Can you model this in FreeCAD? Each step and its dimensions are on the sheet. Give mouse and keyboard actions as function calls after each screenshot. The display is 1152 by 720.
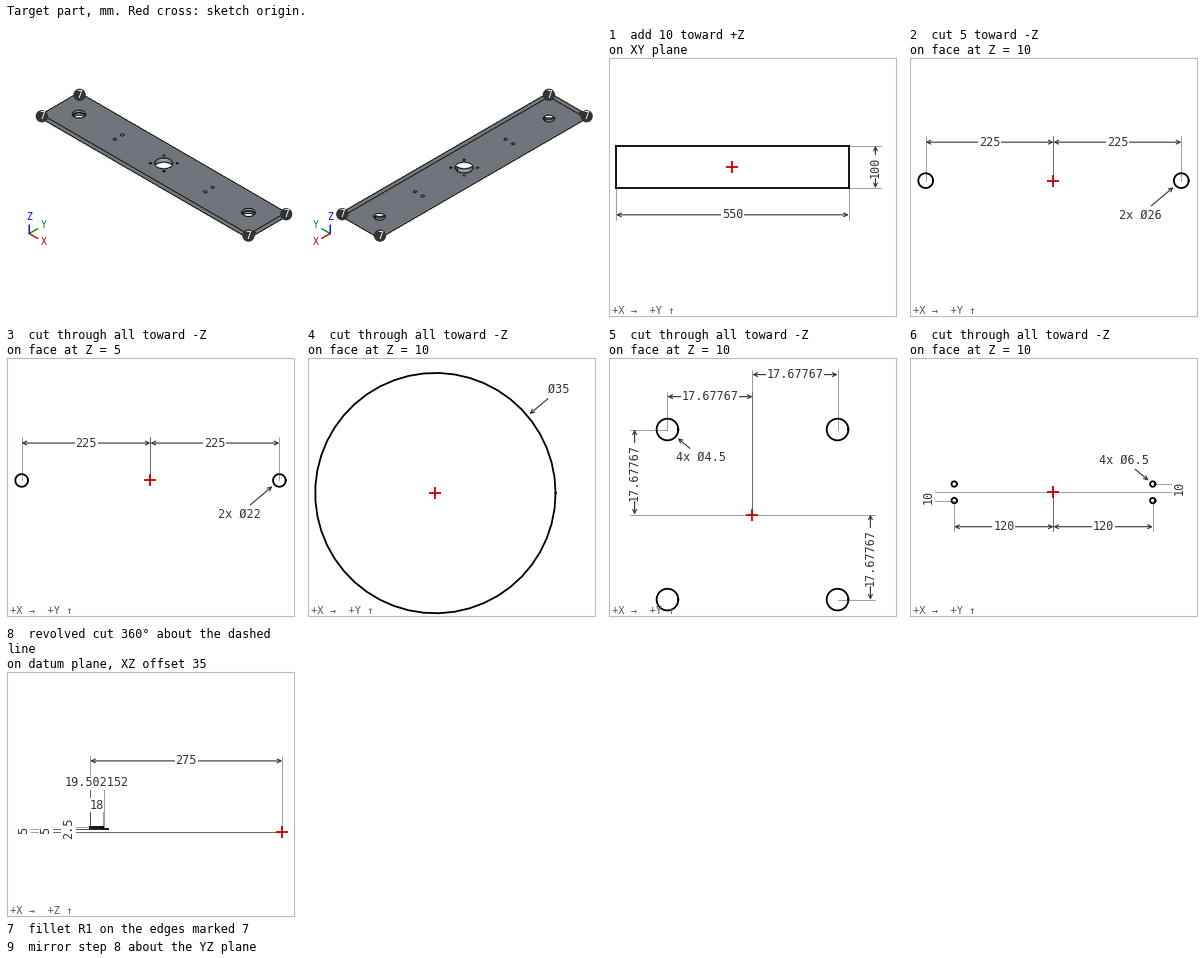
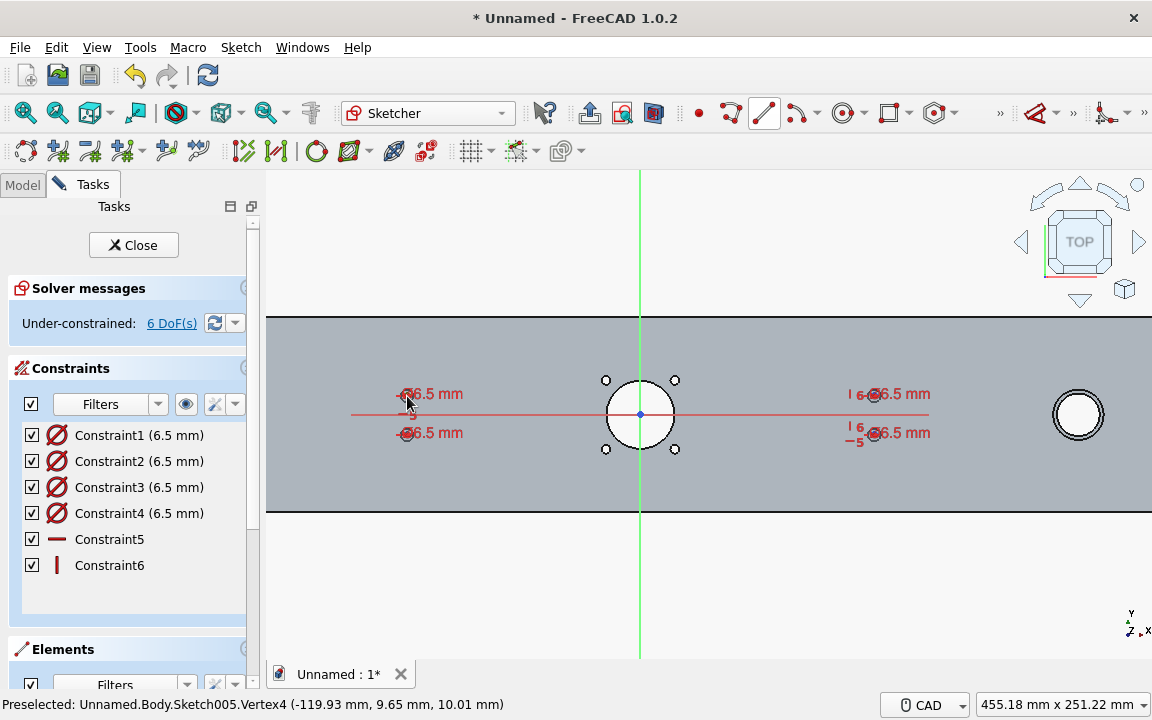
key(v)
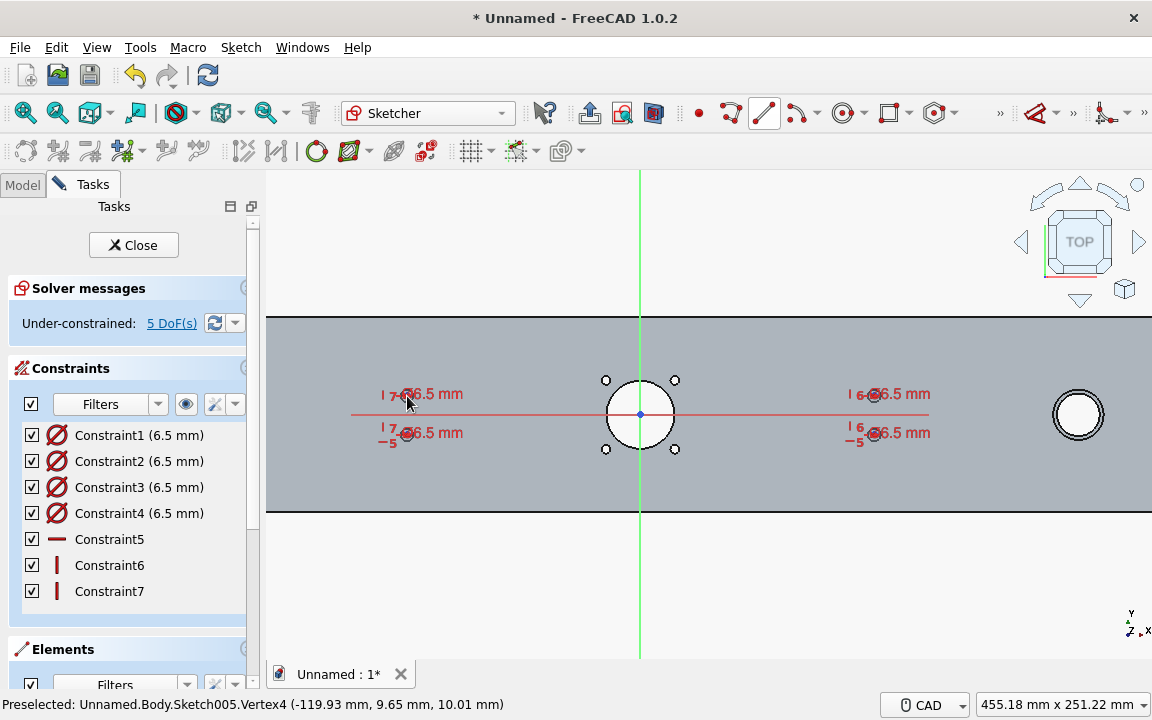
click(874, 396)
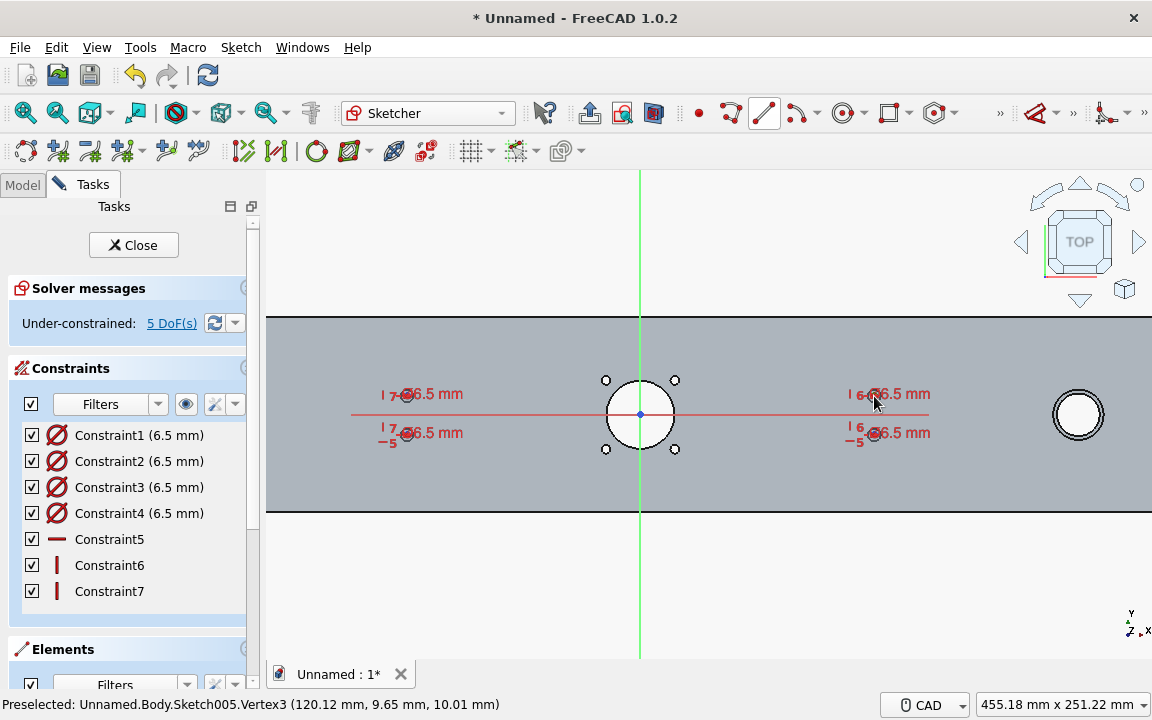
click(407, 396)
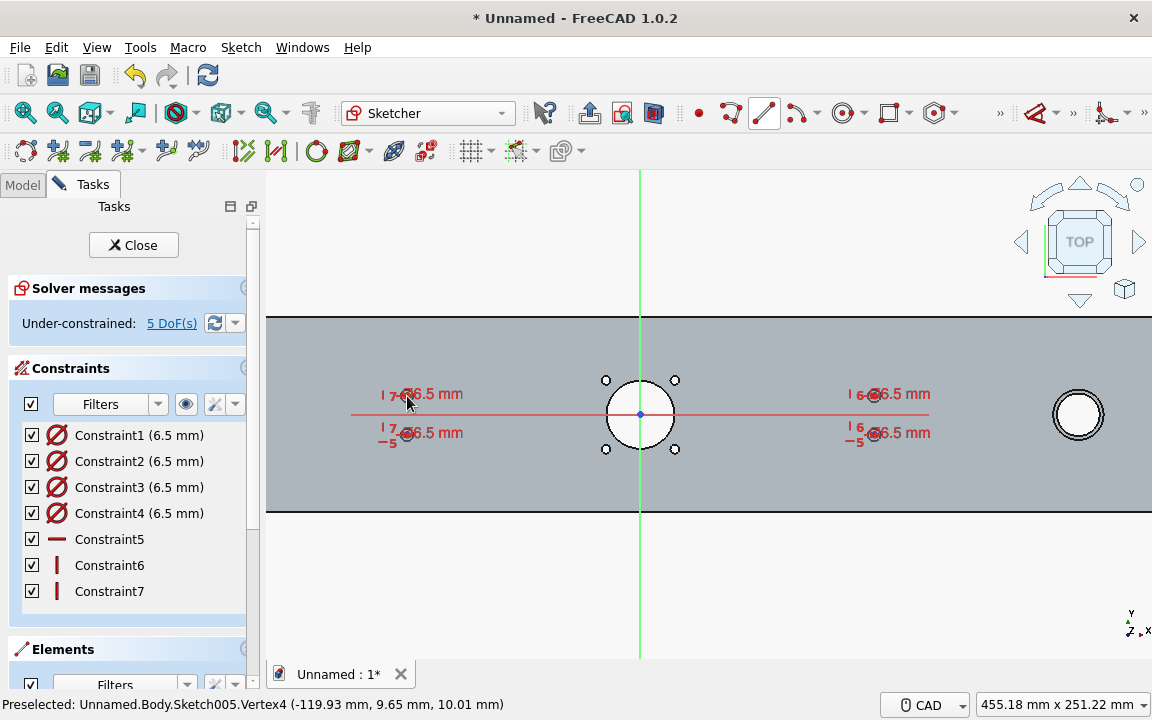
key(h)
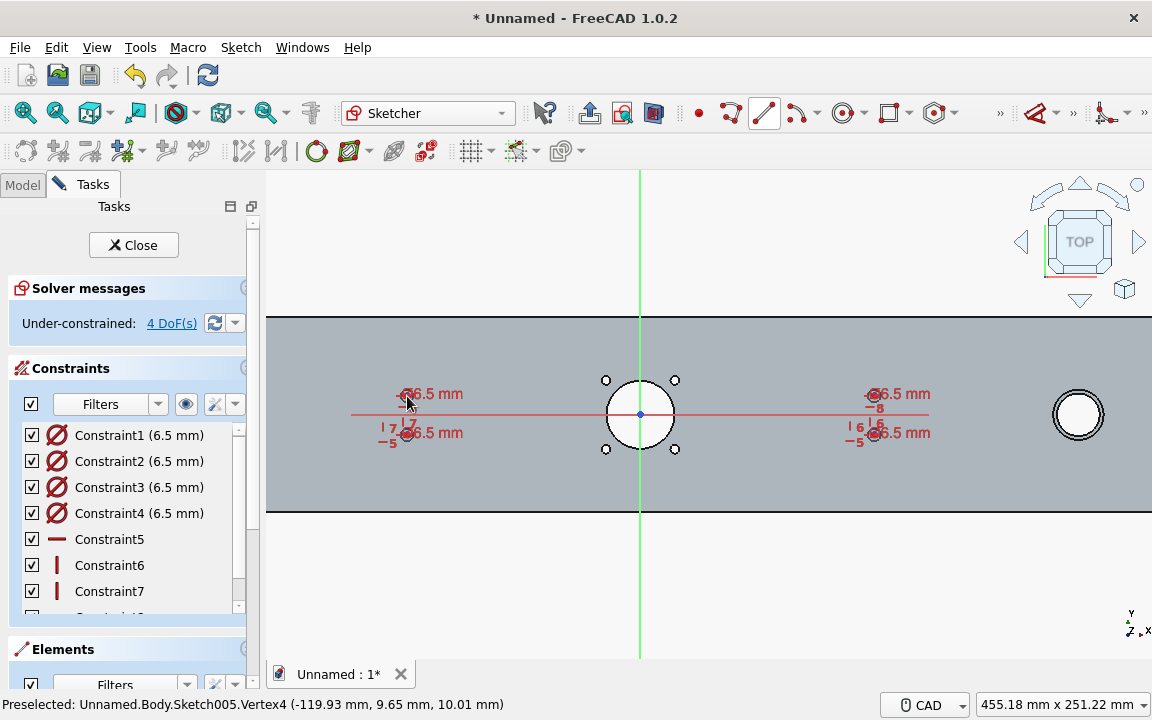
click(1036, 114)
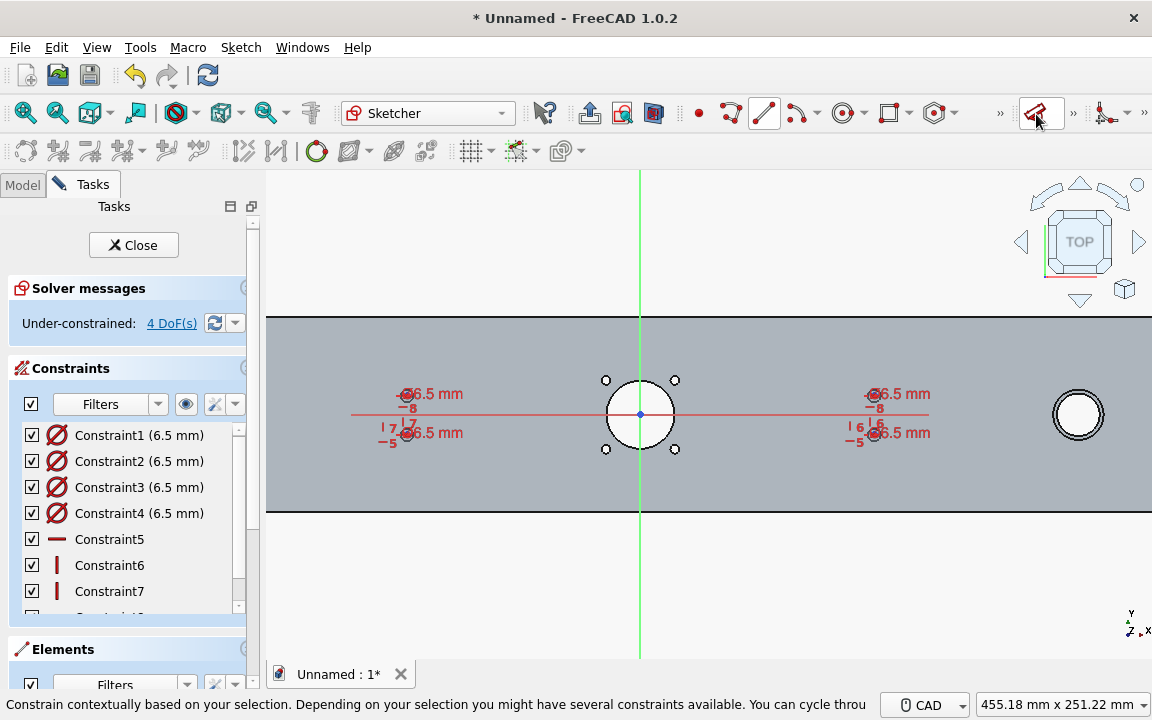
scroll(407, 435, up, 4)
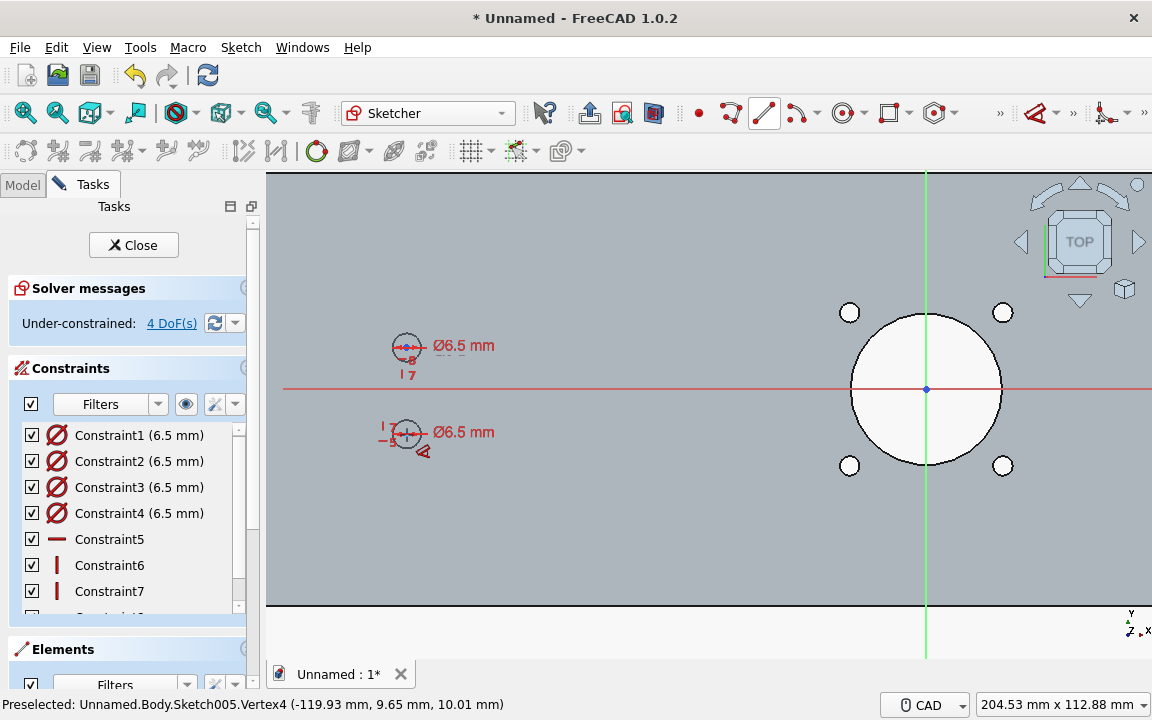
click(407, 434)
click(373, 412)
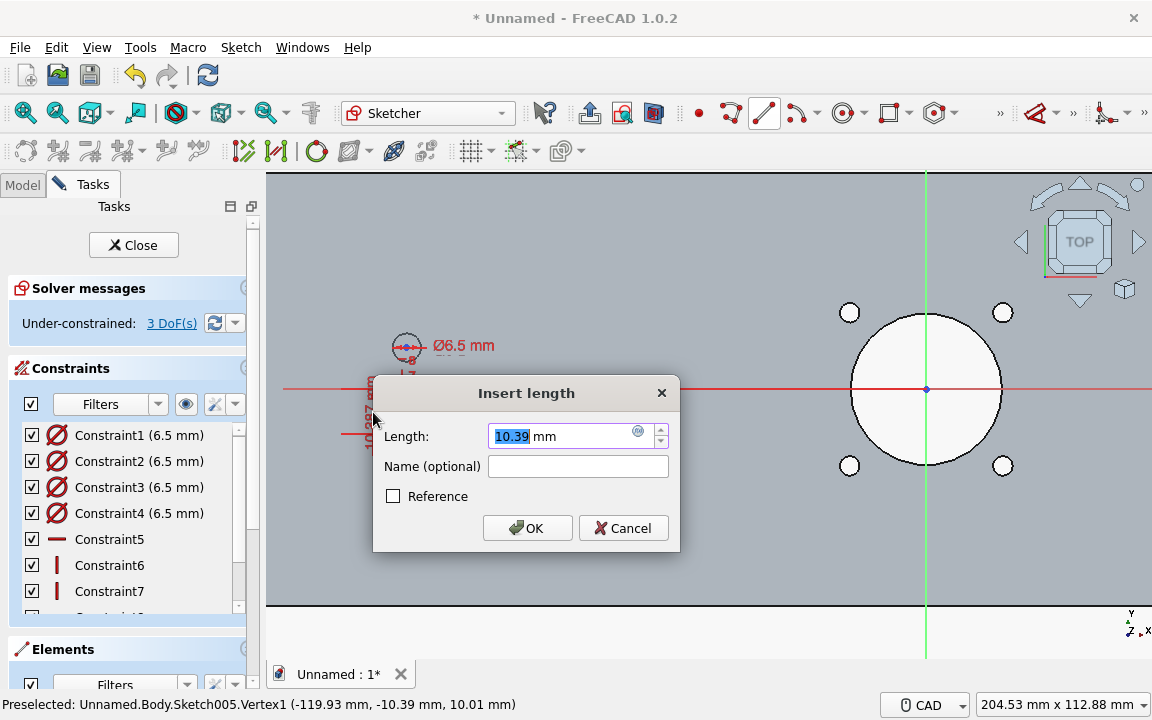
text(10)
key(Return)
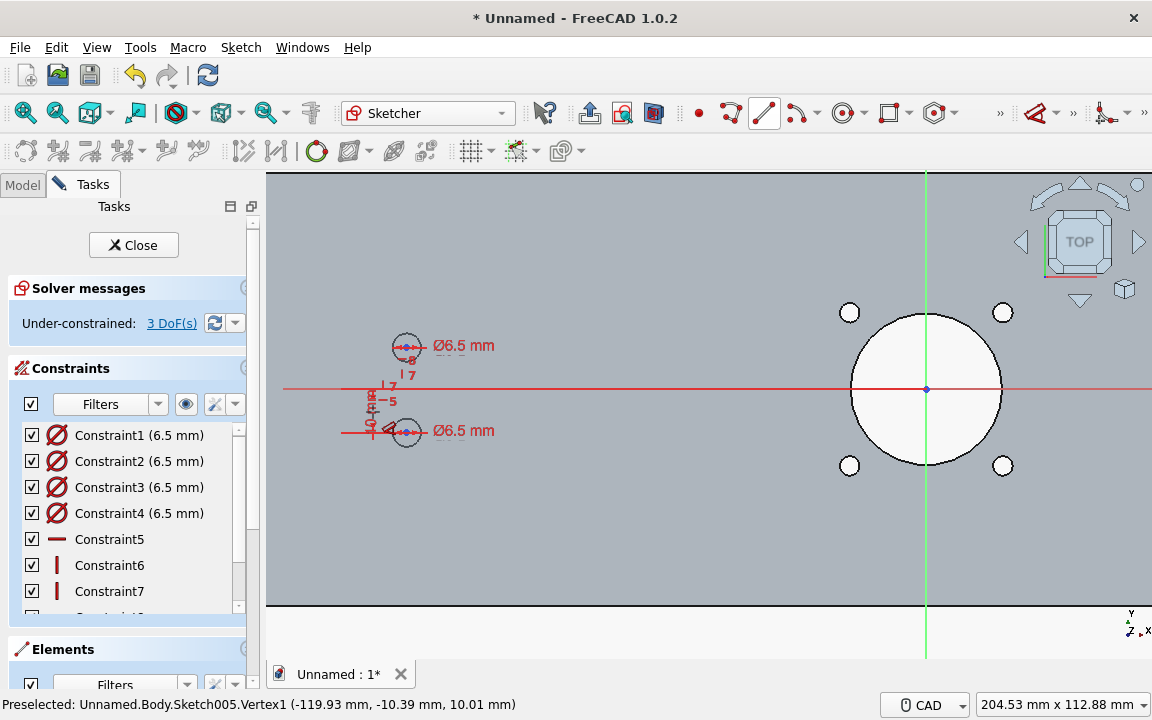
scroll(407, 435, down, 4)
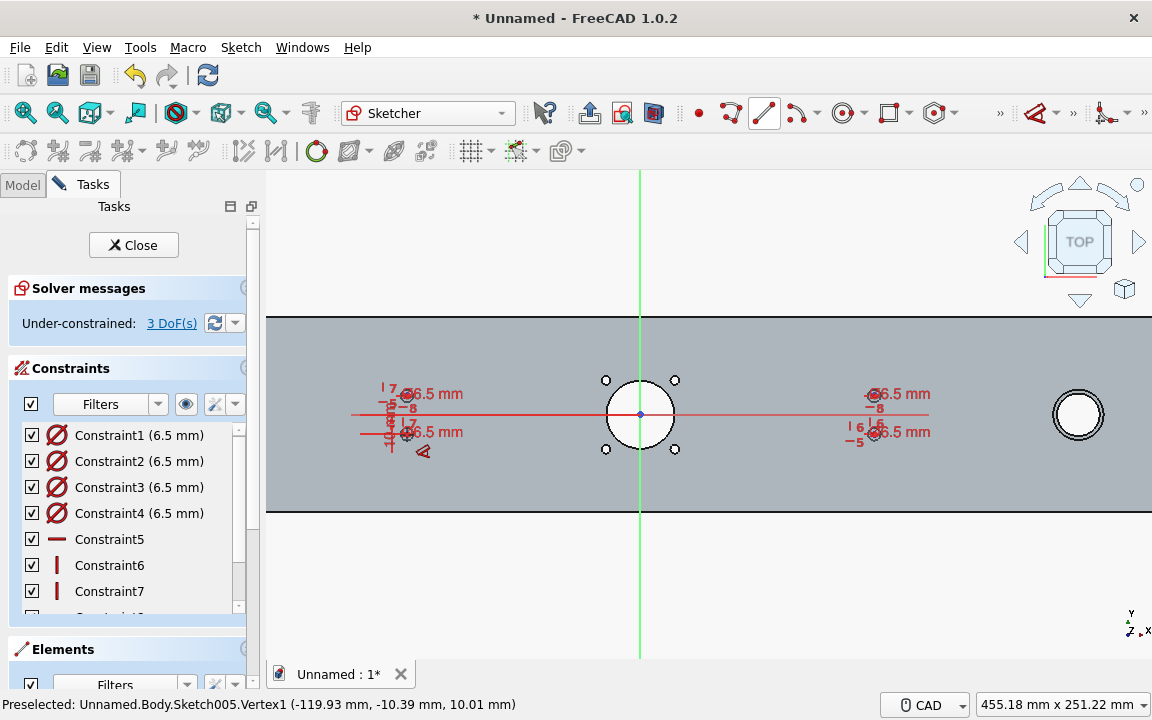
scroll(874, 396, up, 4)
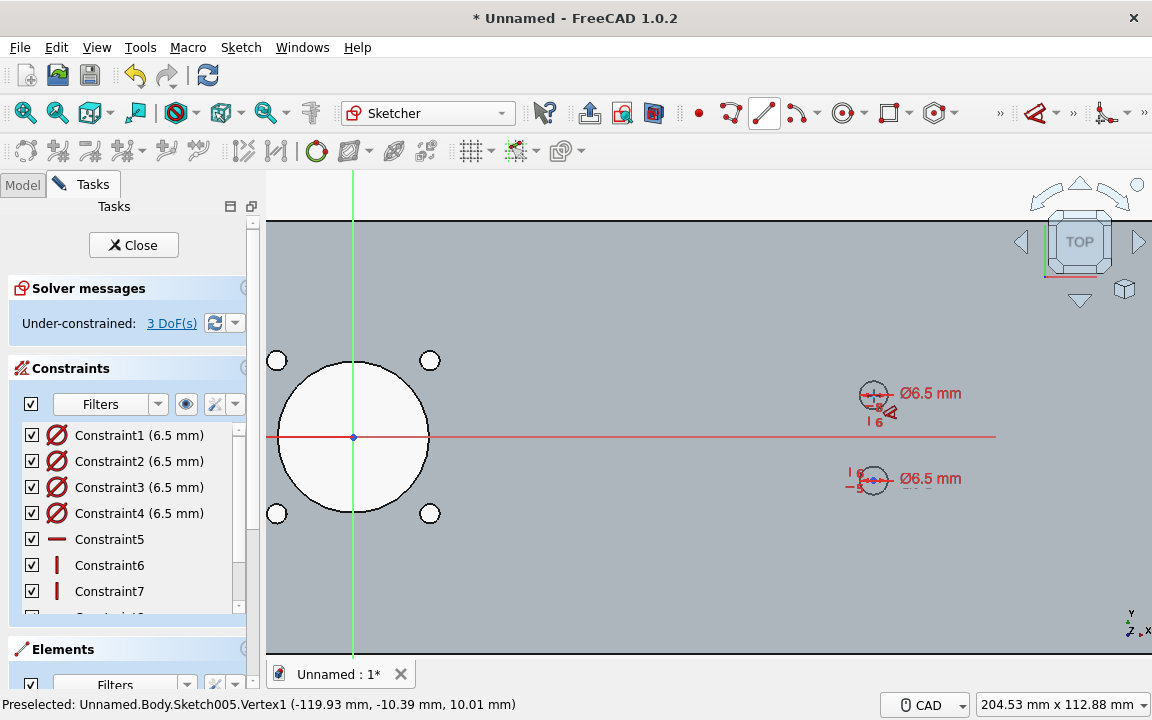
click(874, 395)
click(908, 416)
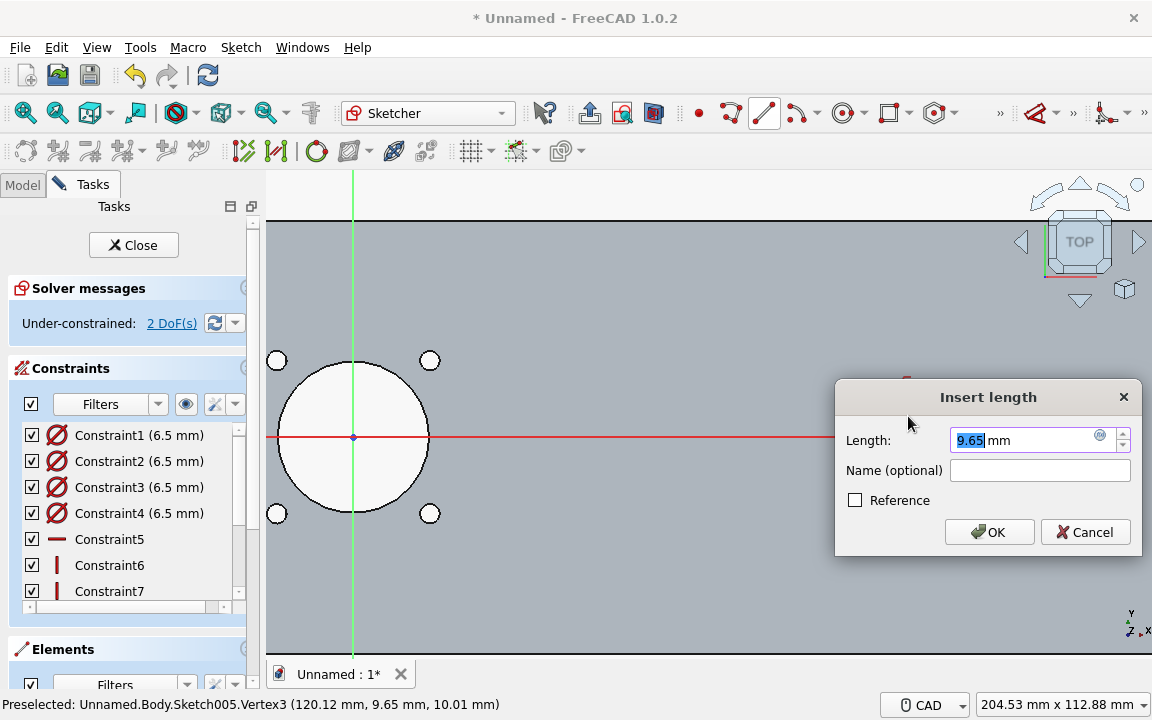
text(10)
key(Return)